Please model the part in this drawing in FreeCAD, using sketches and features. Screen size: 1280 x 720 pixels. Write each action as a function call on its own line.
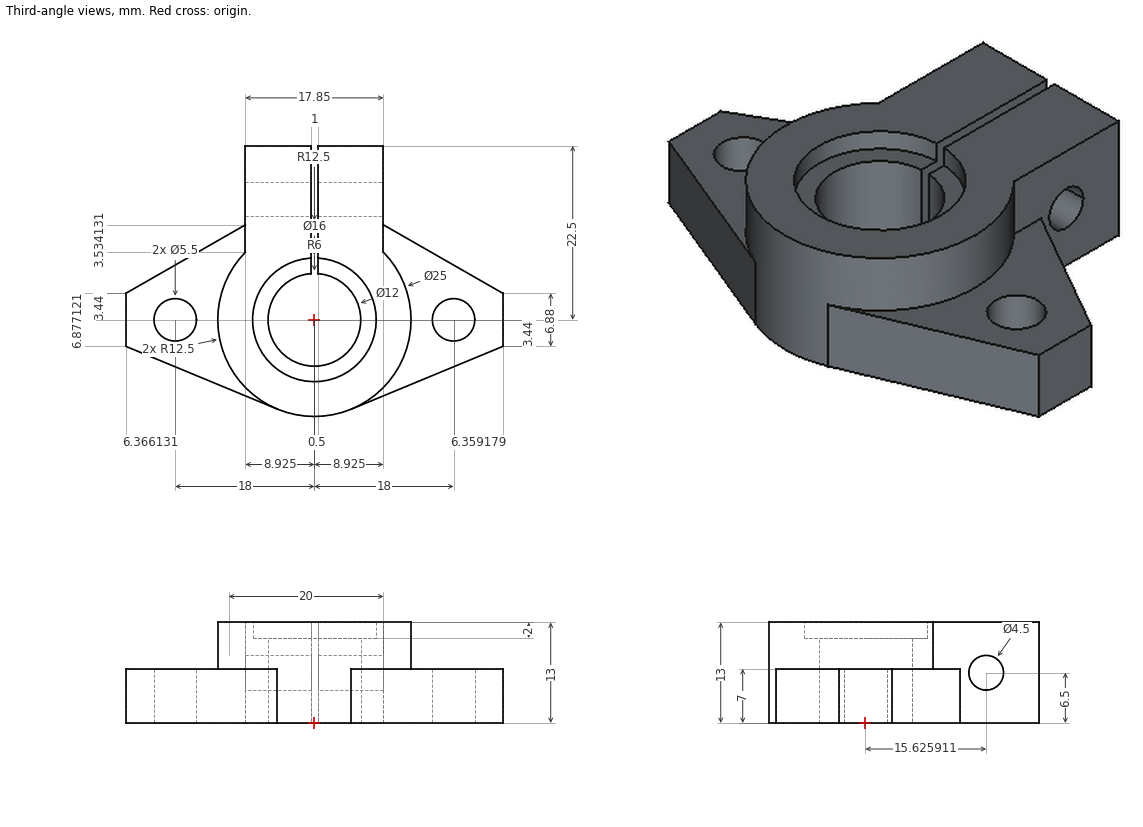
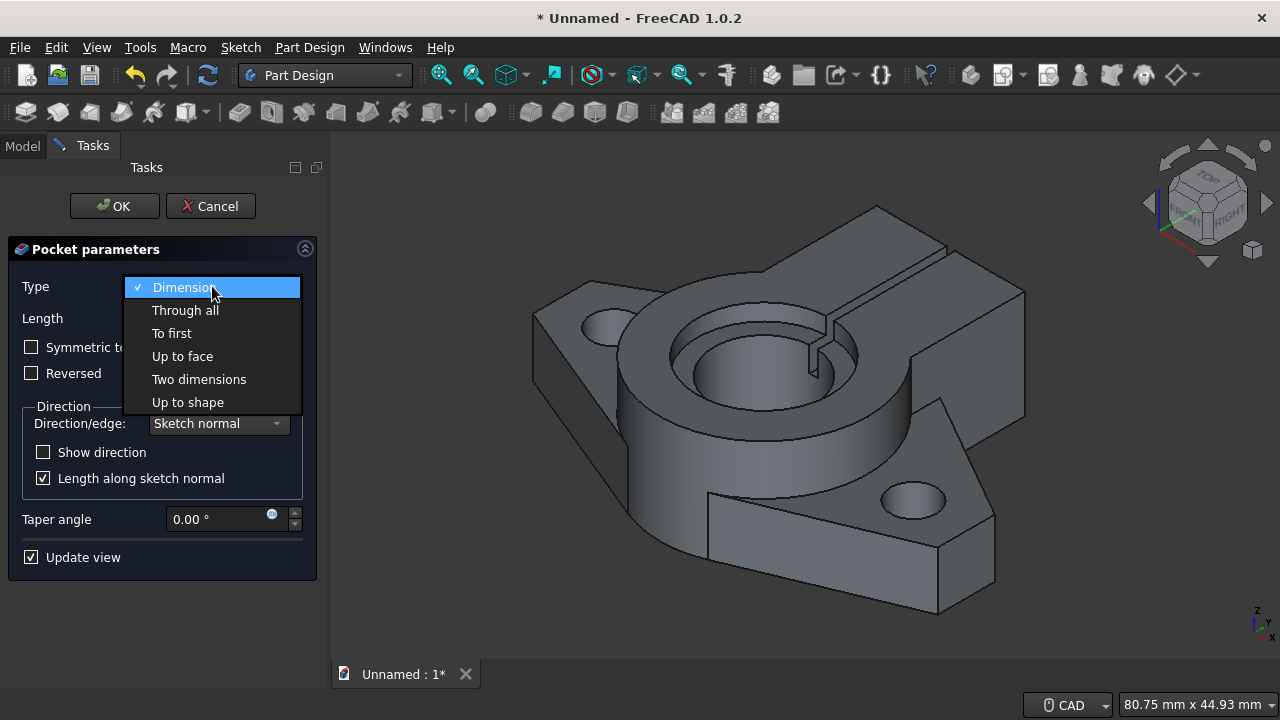
click(212, 310)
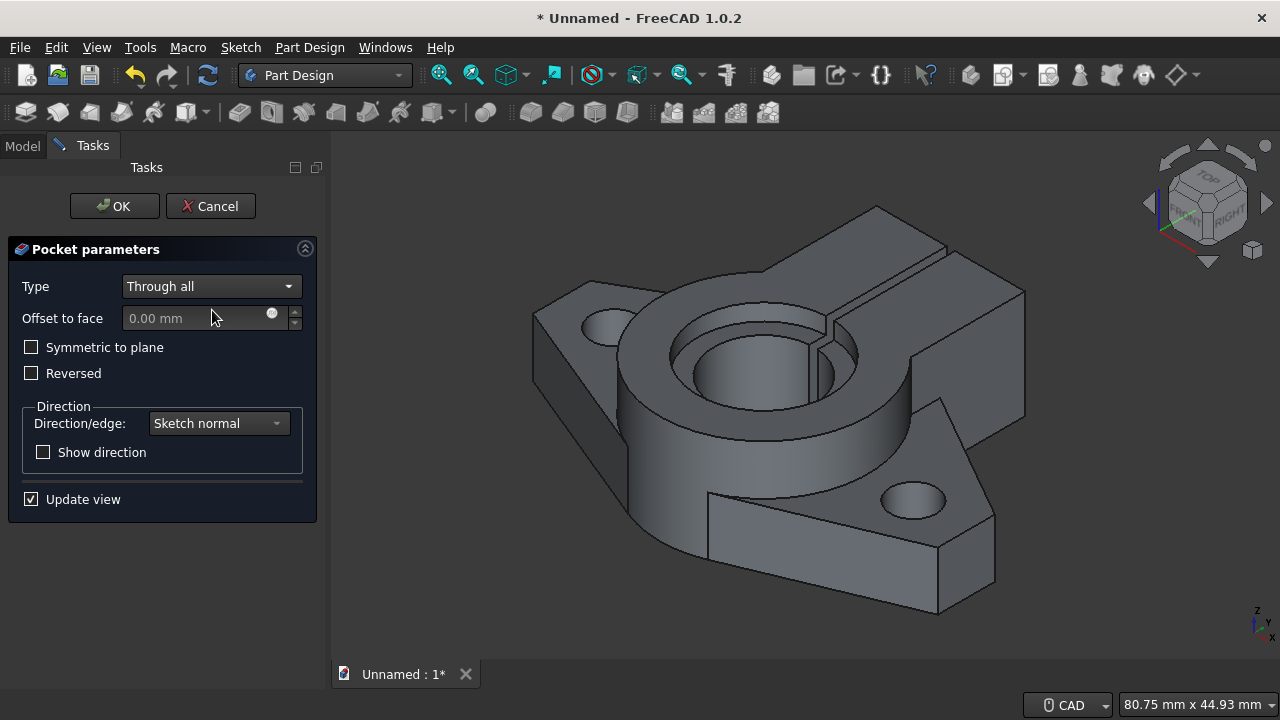
click(115, 206)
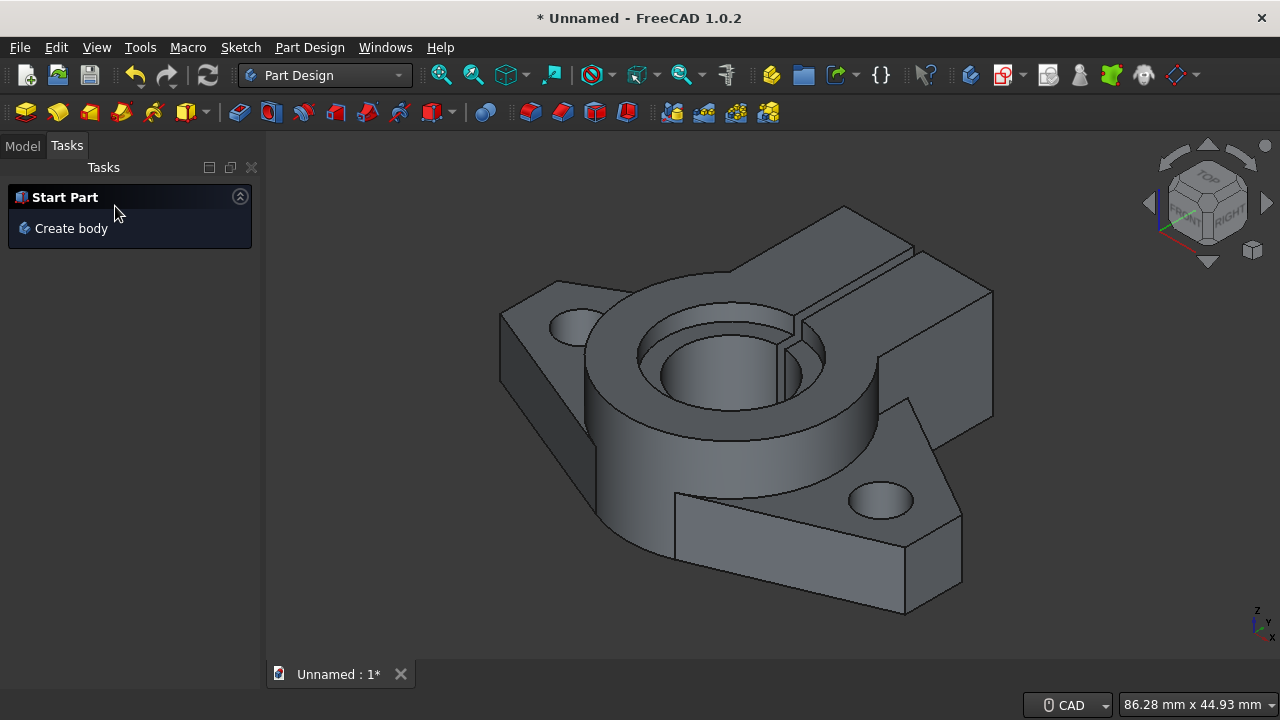
click(952, 376)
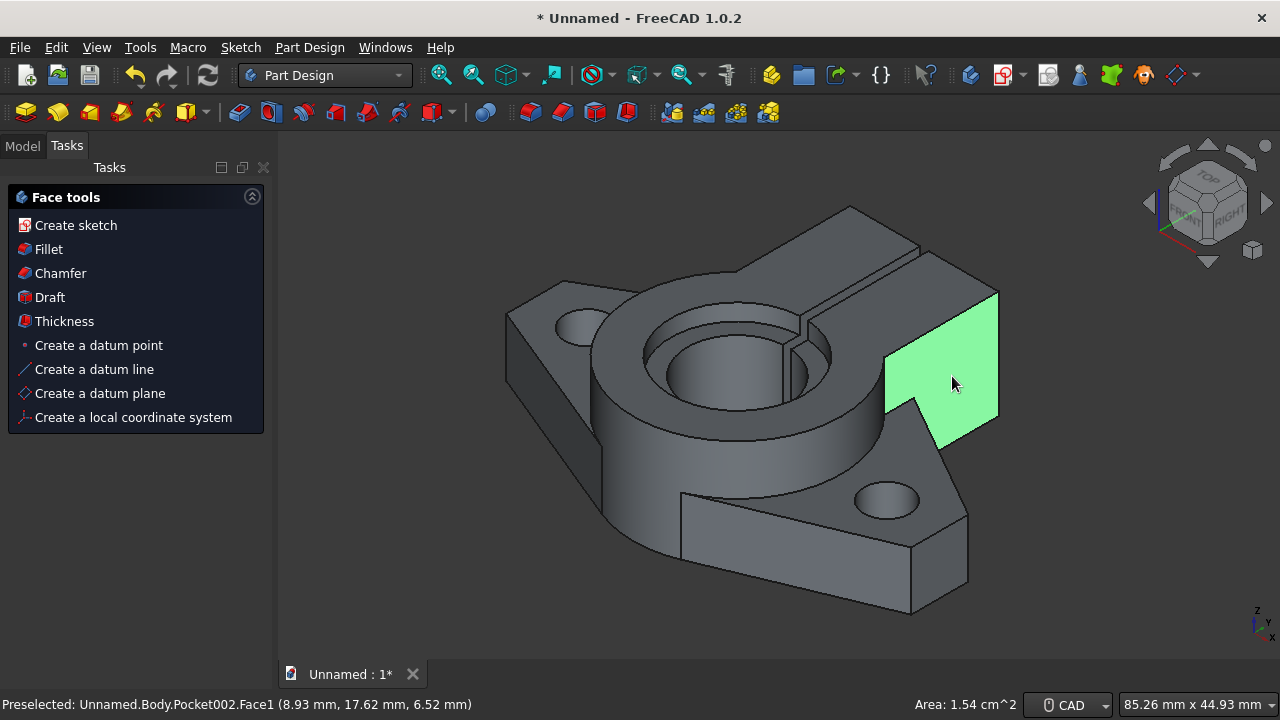
click(1004, 76)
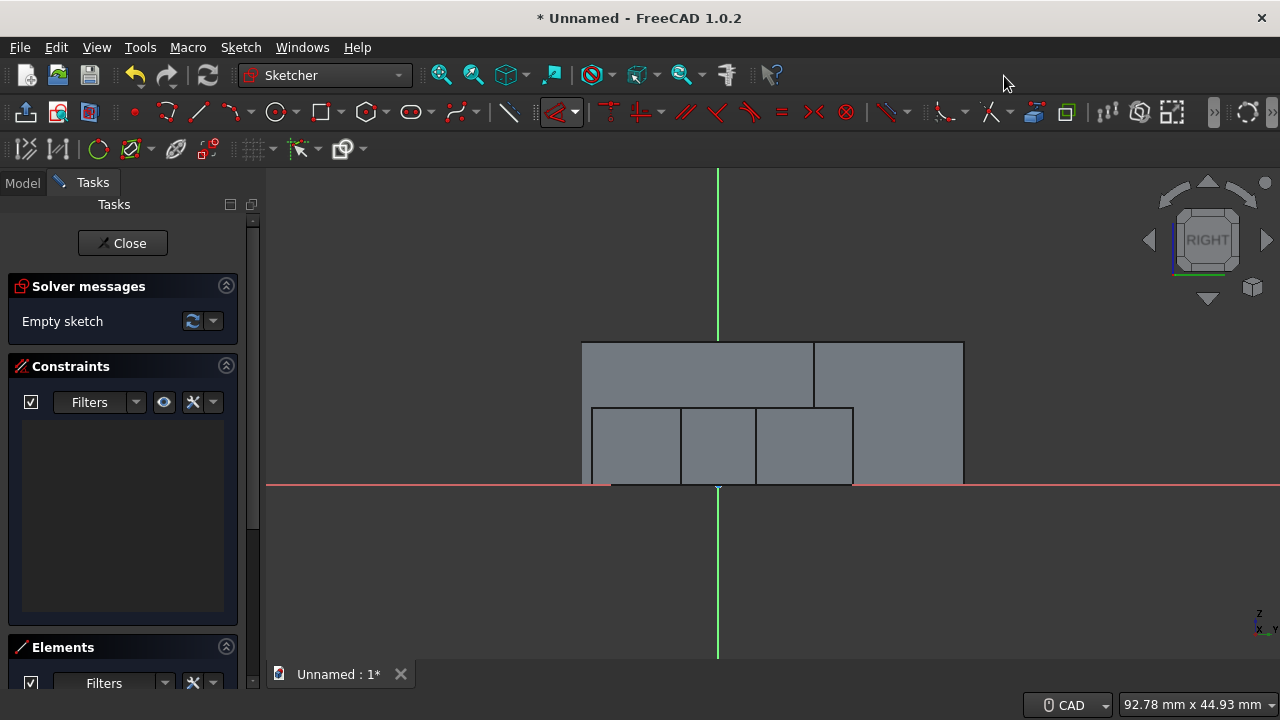
click(90, 112)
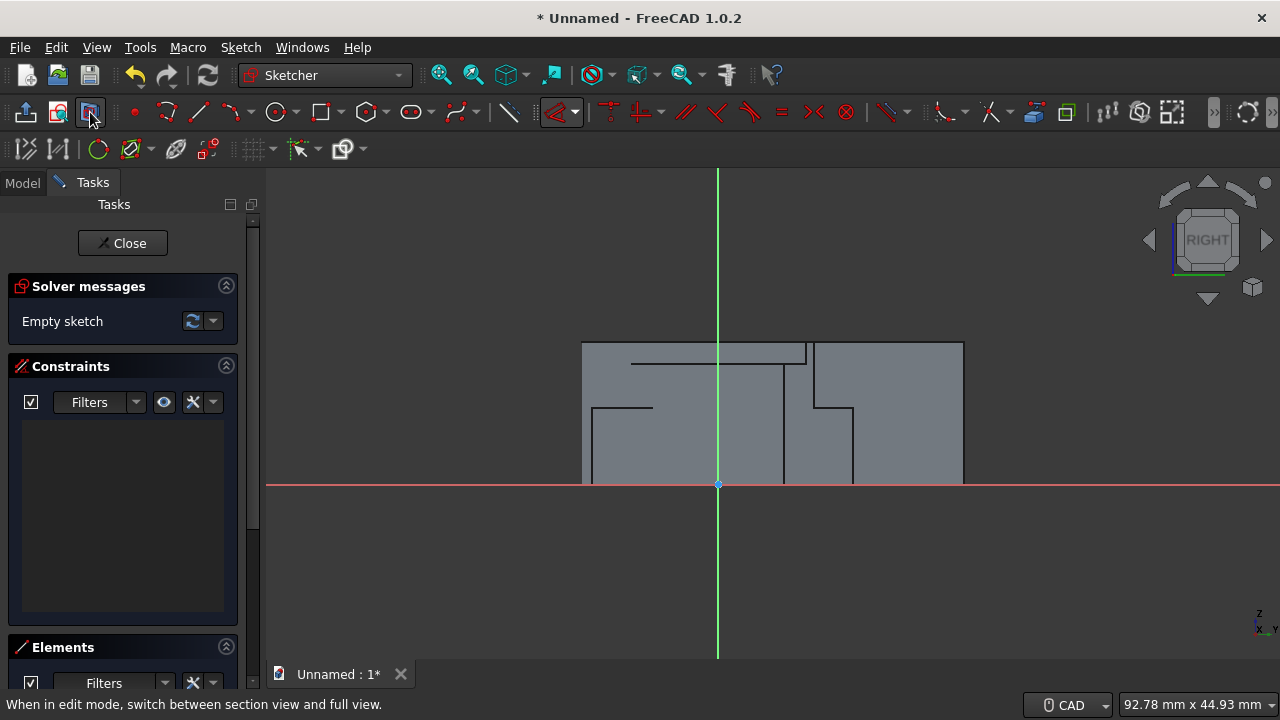
scroll(926, 413, up, 9)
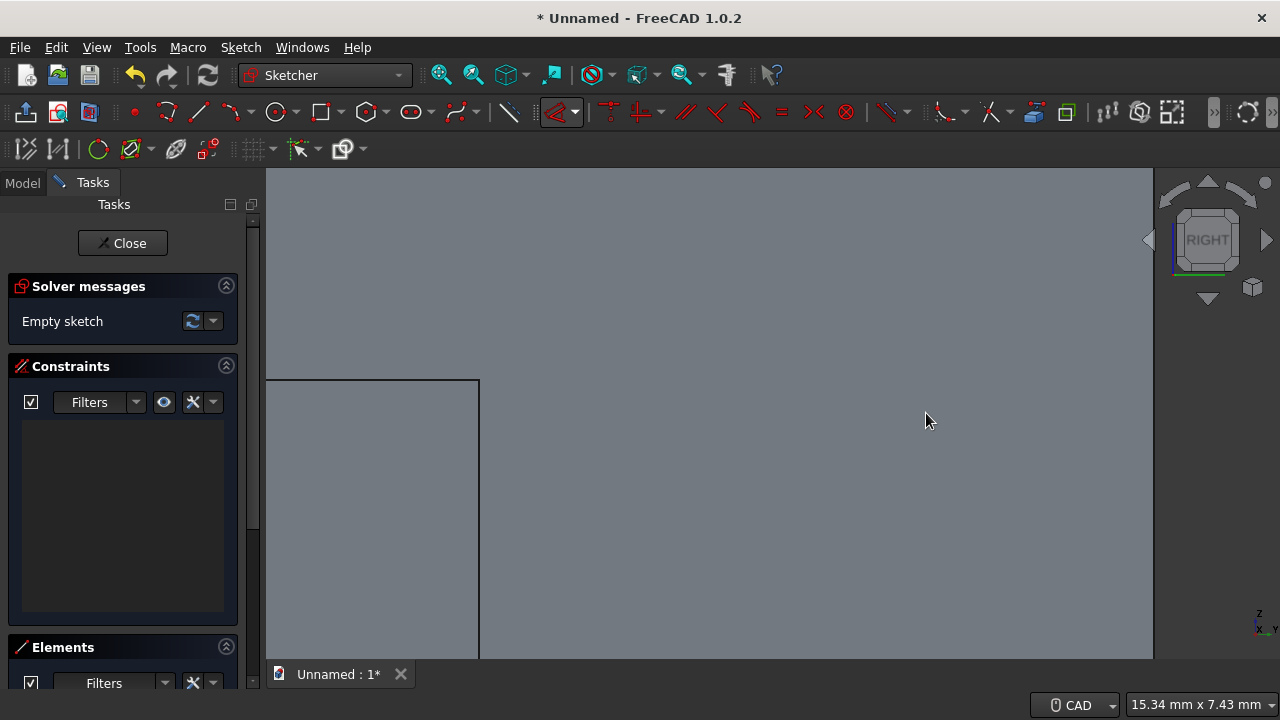
click(276, 112)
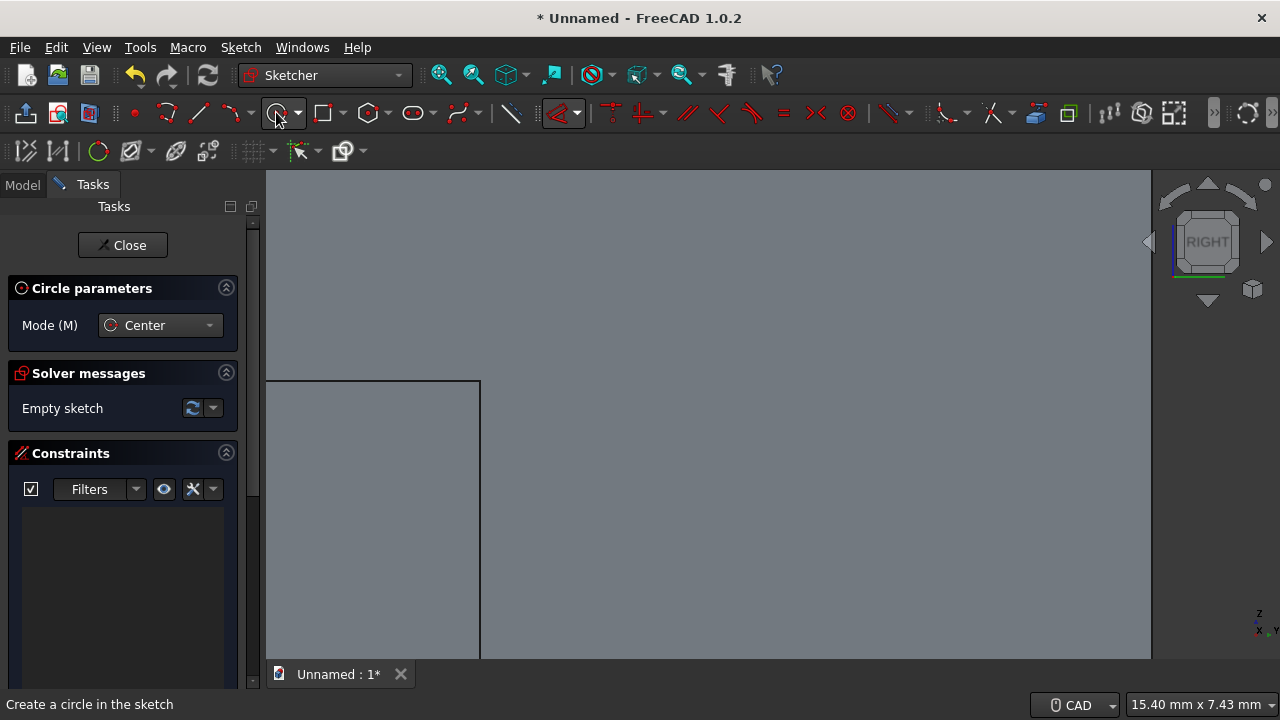
click(700, 414)
click(804, 310)
key(Escape)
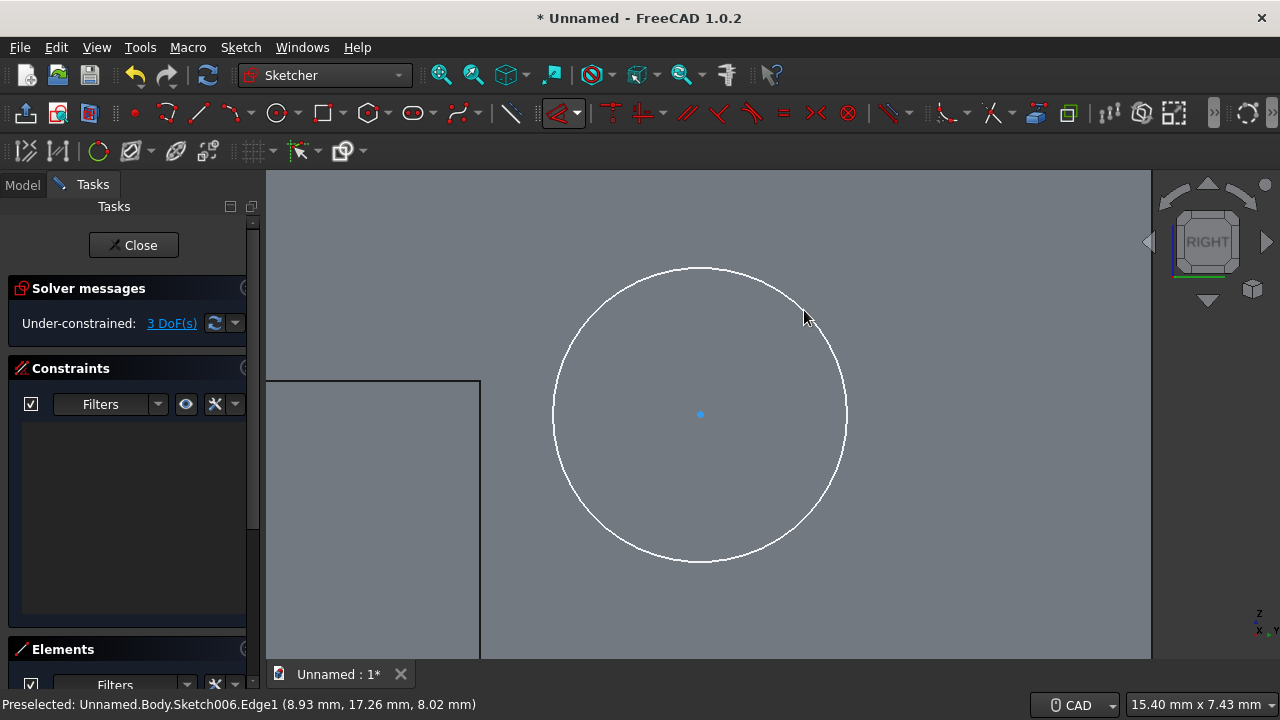
click(804, 311)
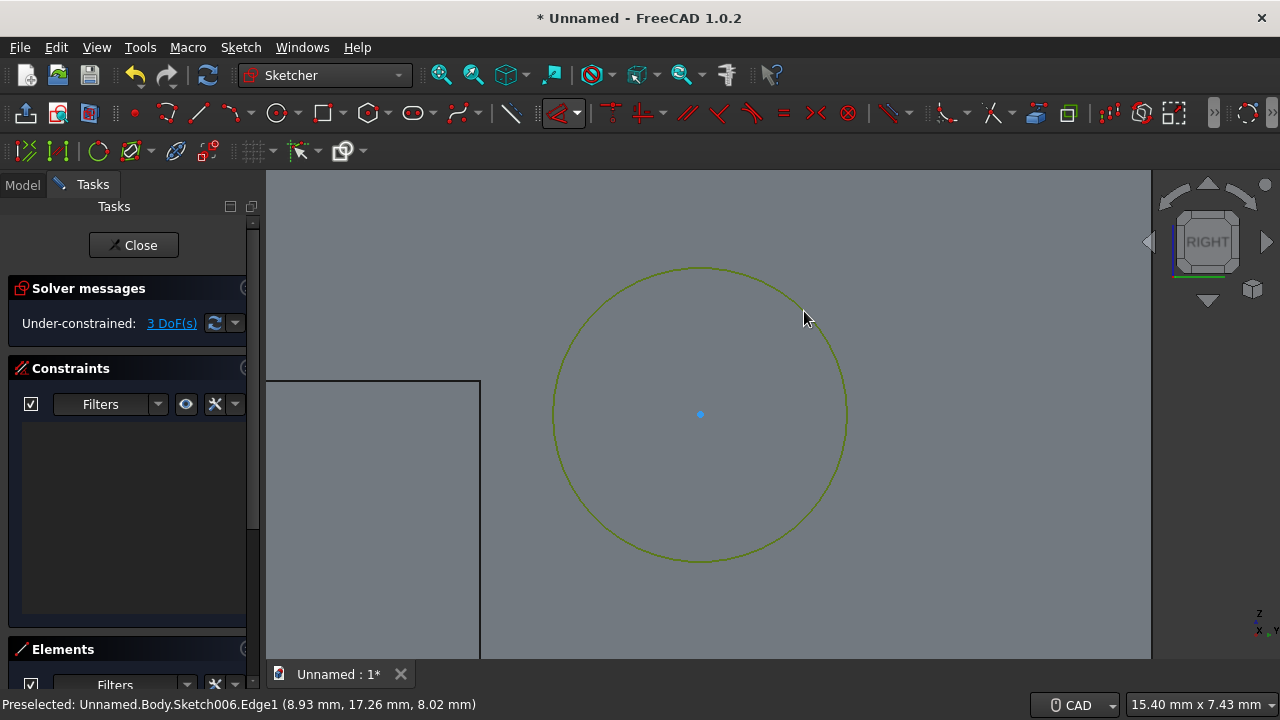
key(k)
key(o)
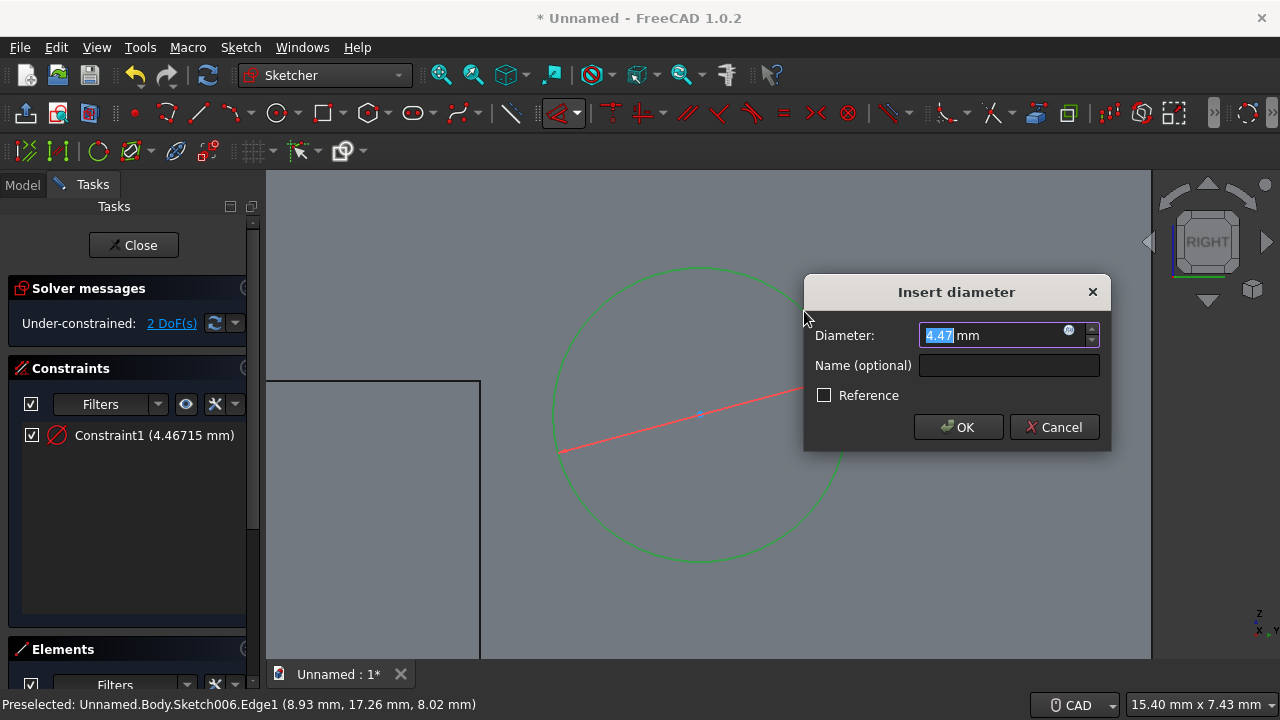
text(4.5)
key(Return)